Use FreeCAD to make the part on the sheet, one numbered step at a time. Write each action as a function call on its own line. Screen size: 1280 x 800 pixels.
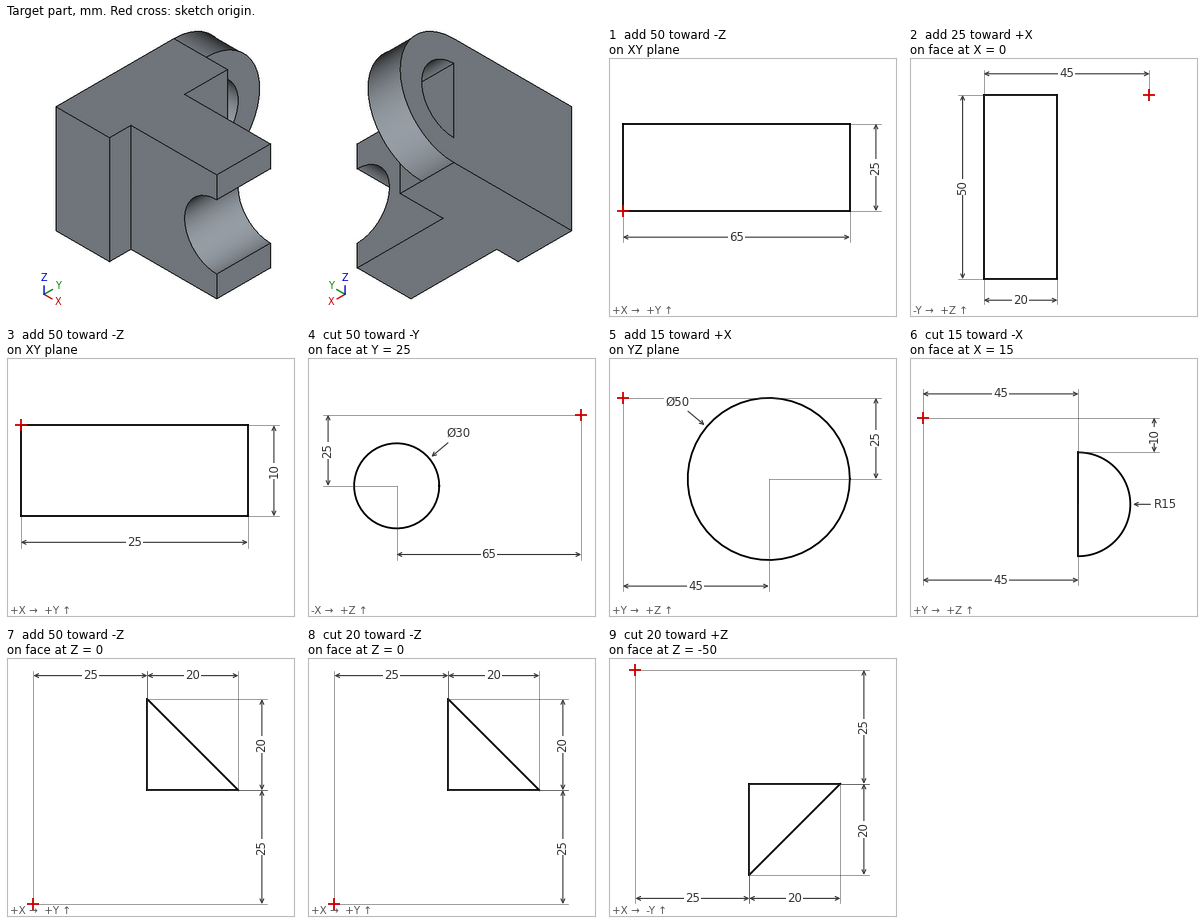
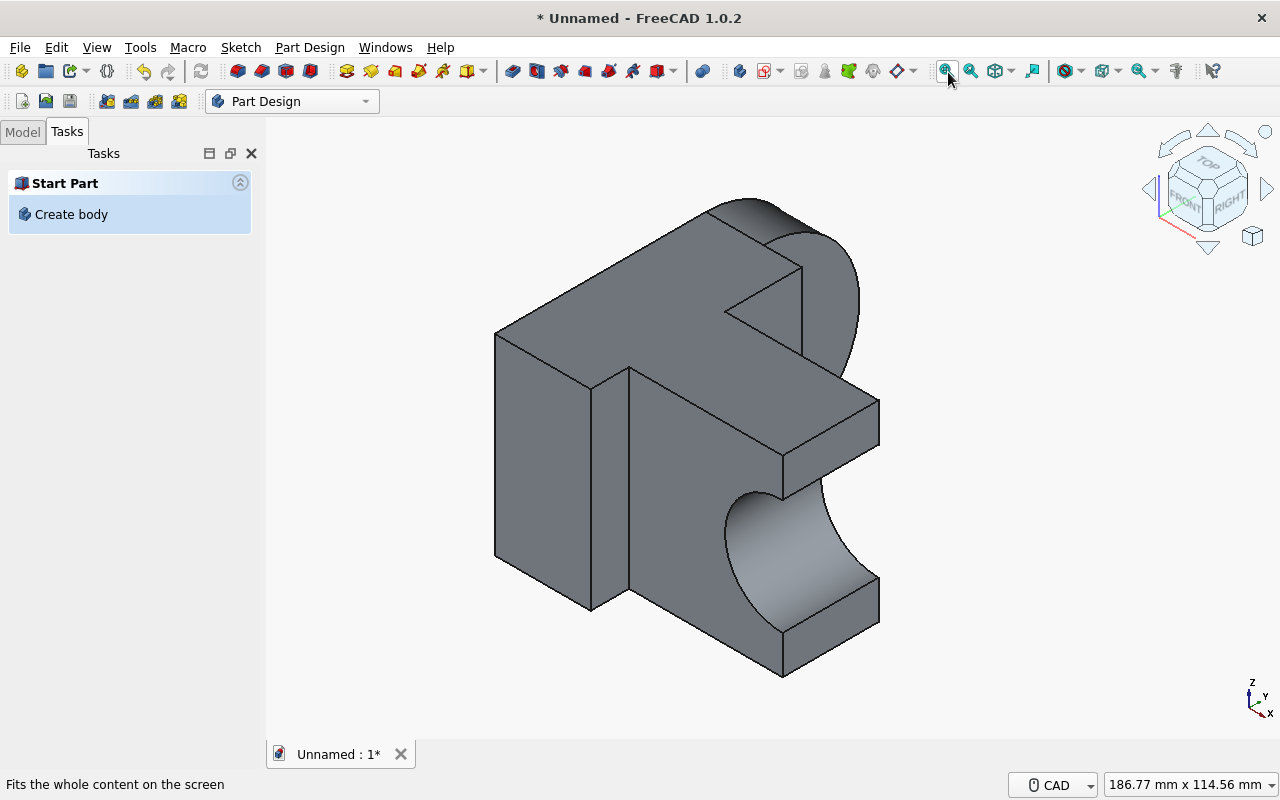
click(811, 327)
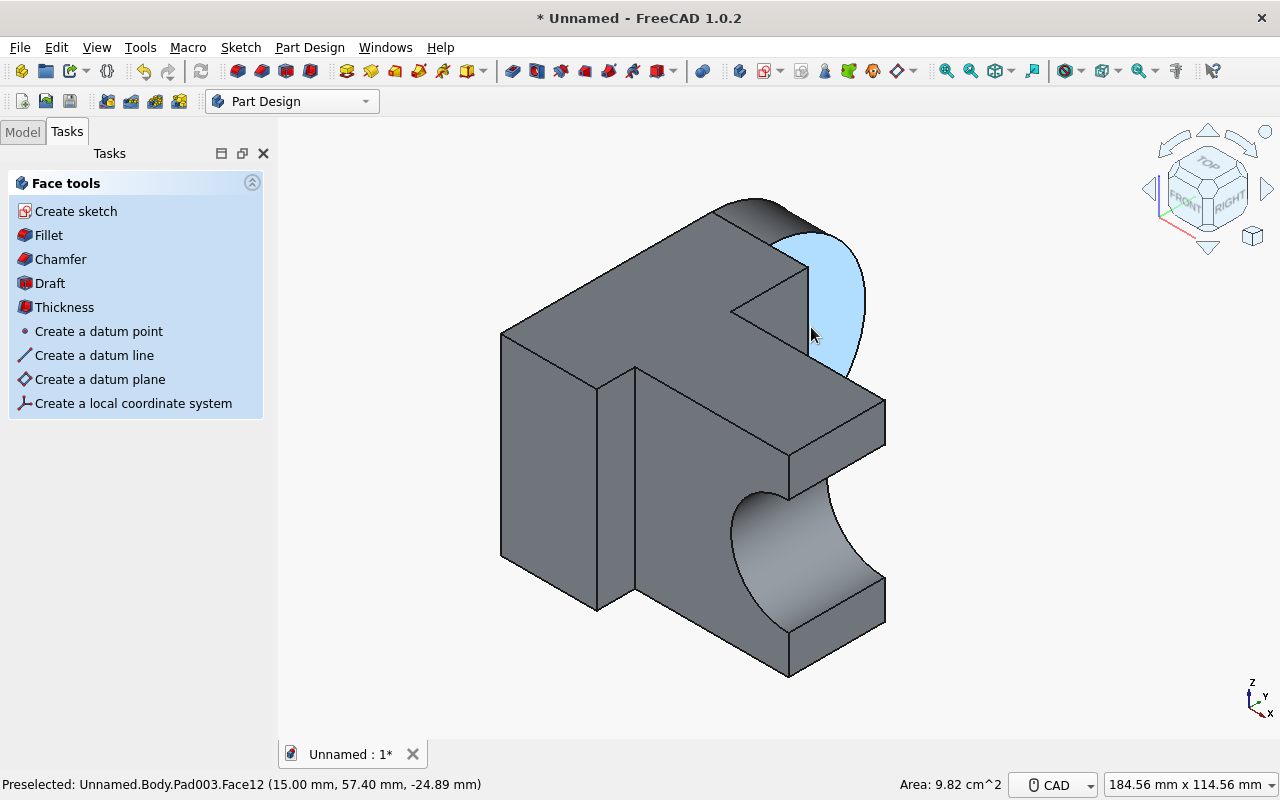
click(764, 72)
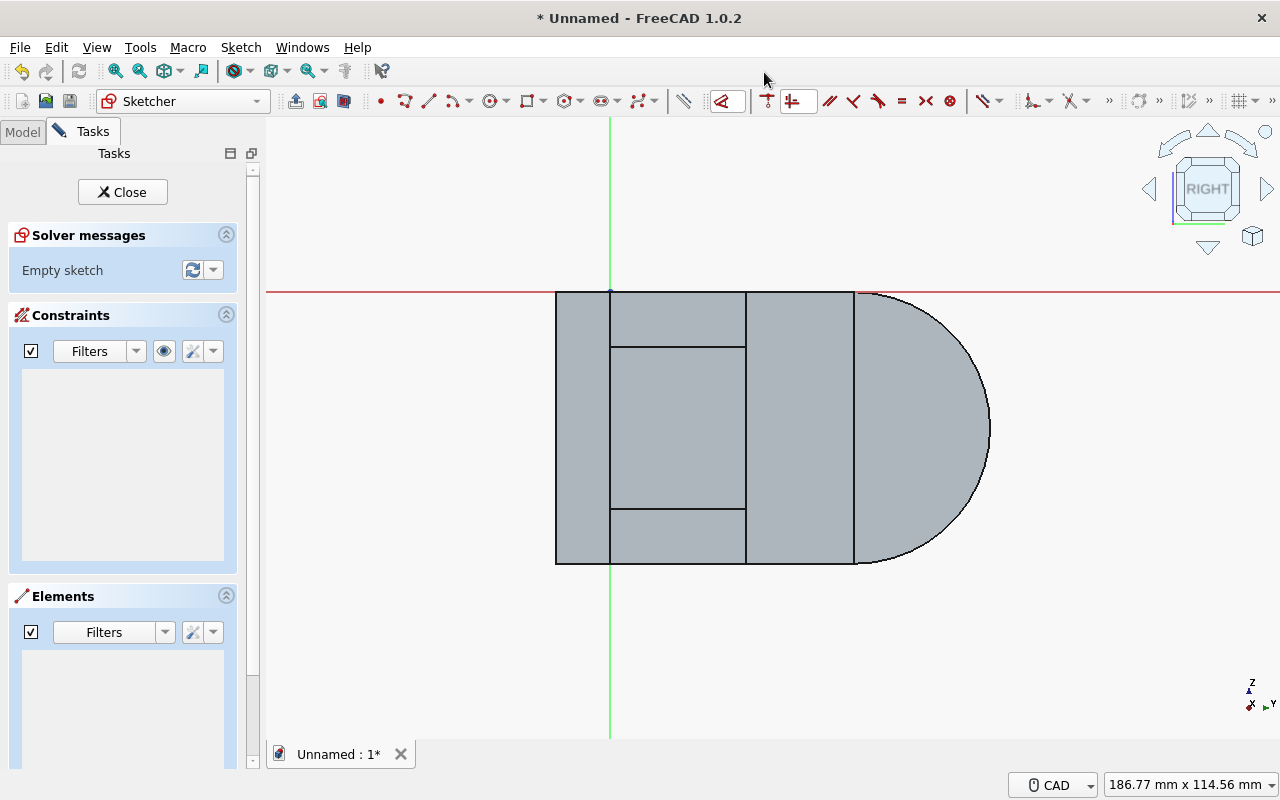
scroll(856, 368, up, 3)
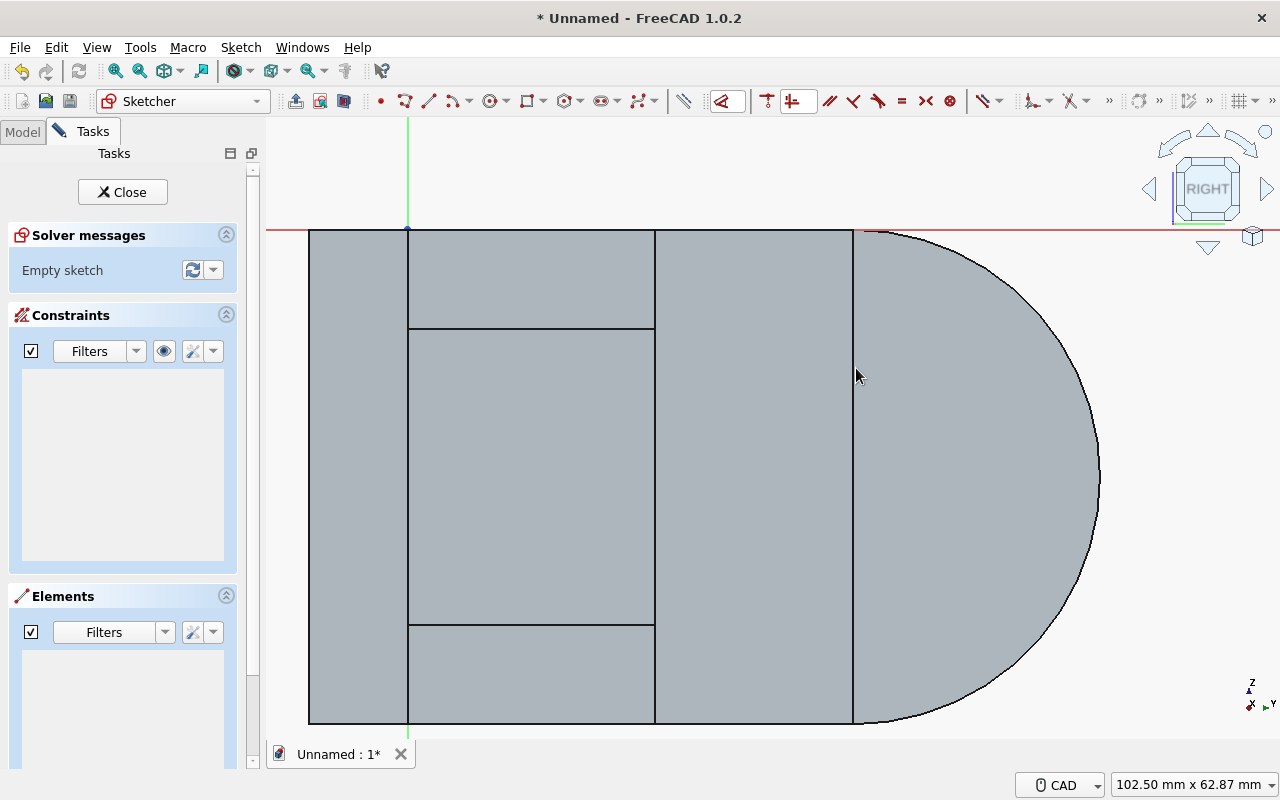
click(430, 102)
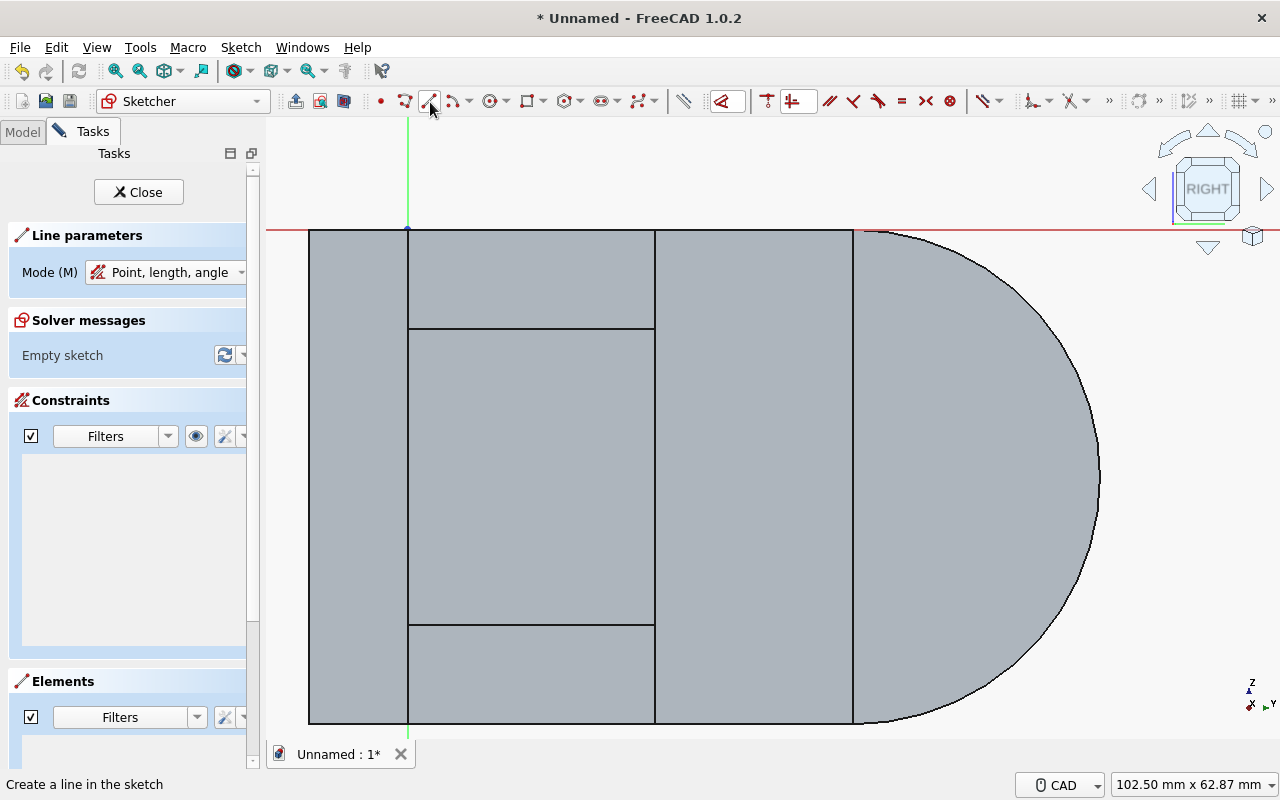
click(853, 329)
click(853, 625)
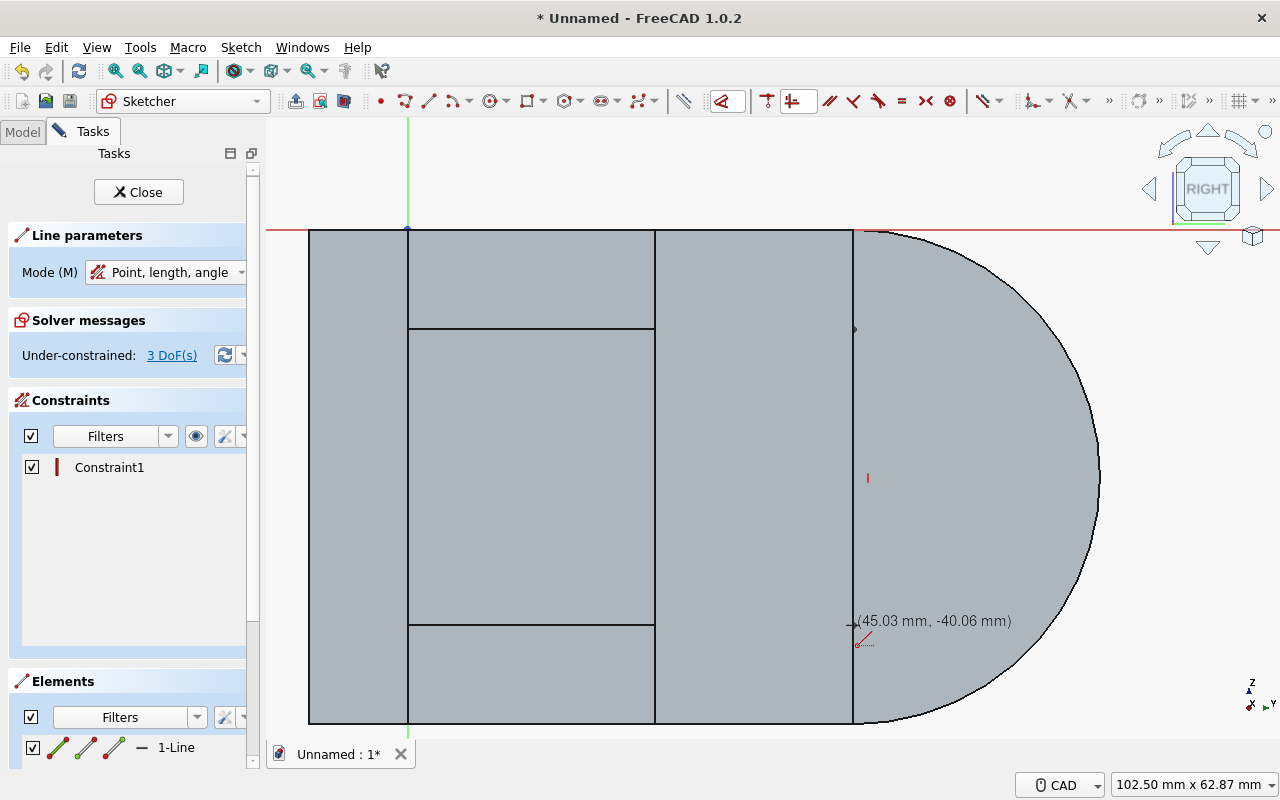
key(g)
key(3)
key(a)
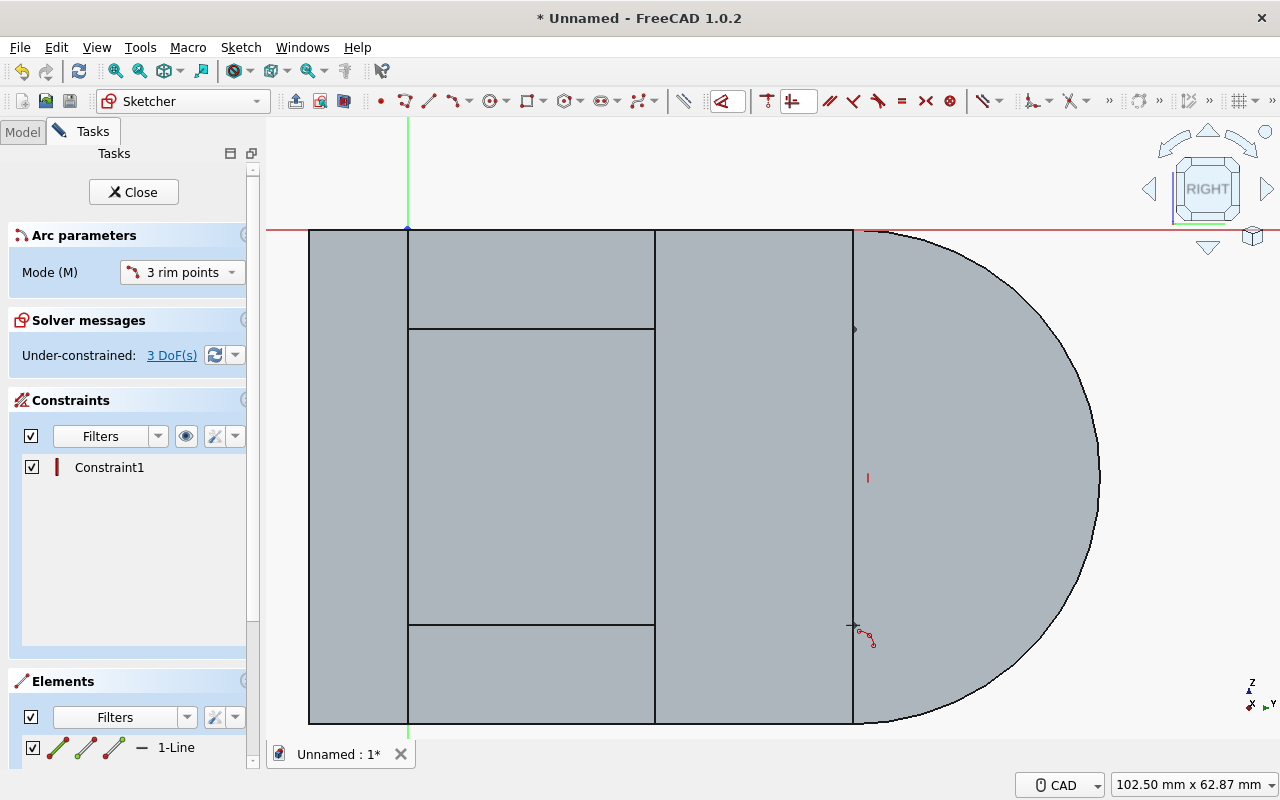
click(853, 626)
click(853, 330)
click(1001, 477)
key(Escape)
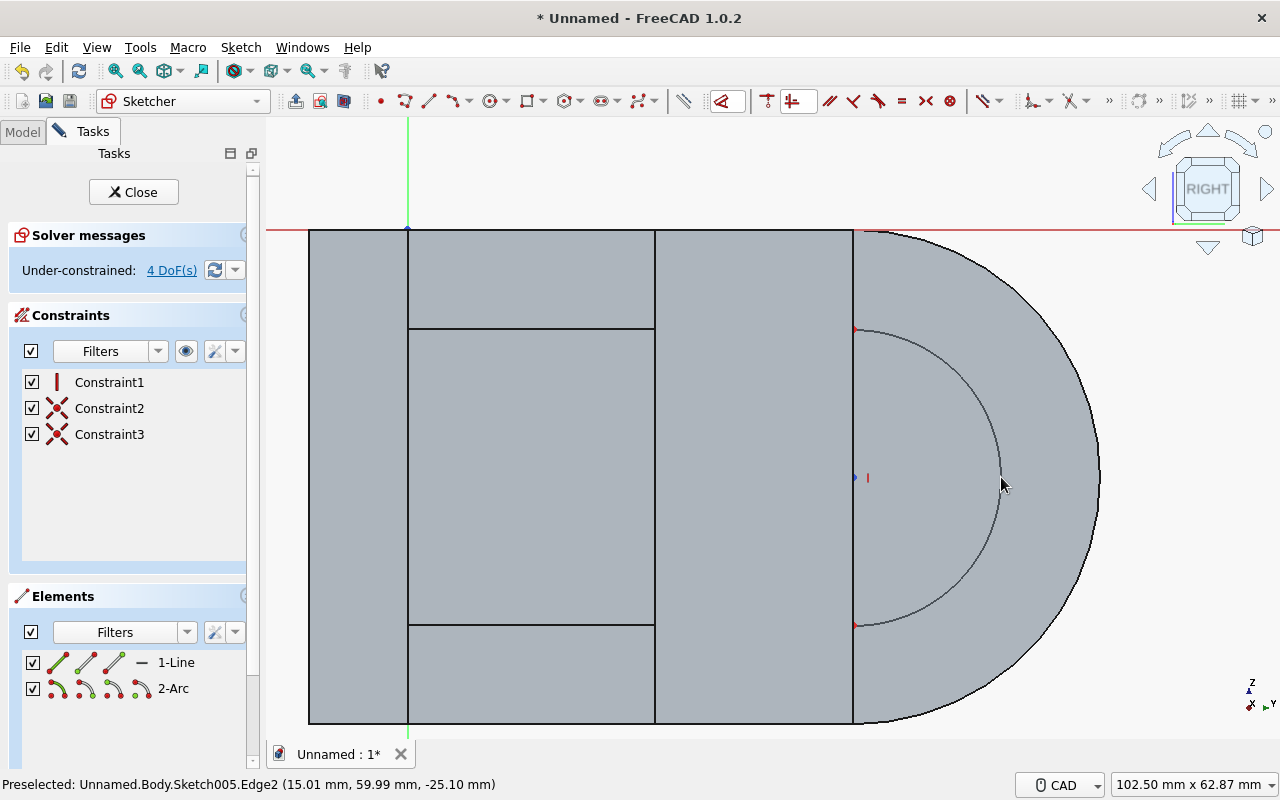
click(973, 565)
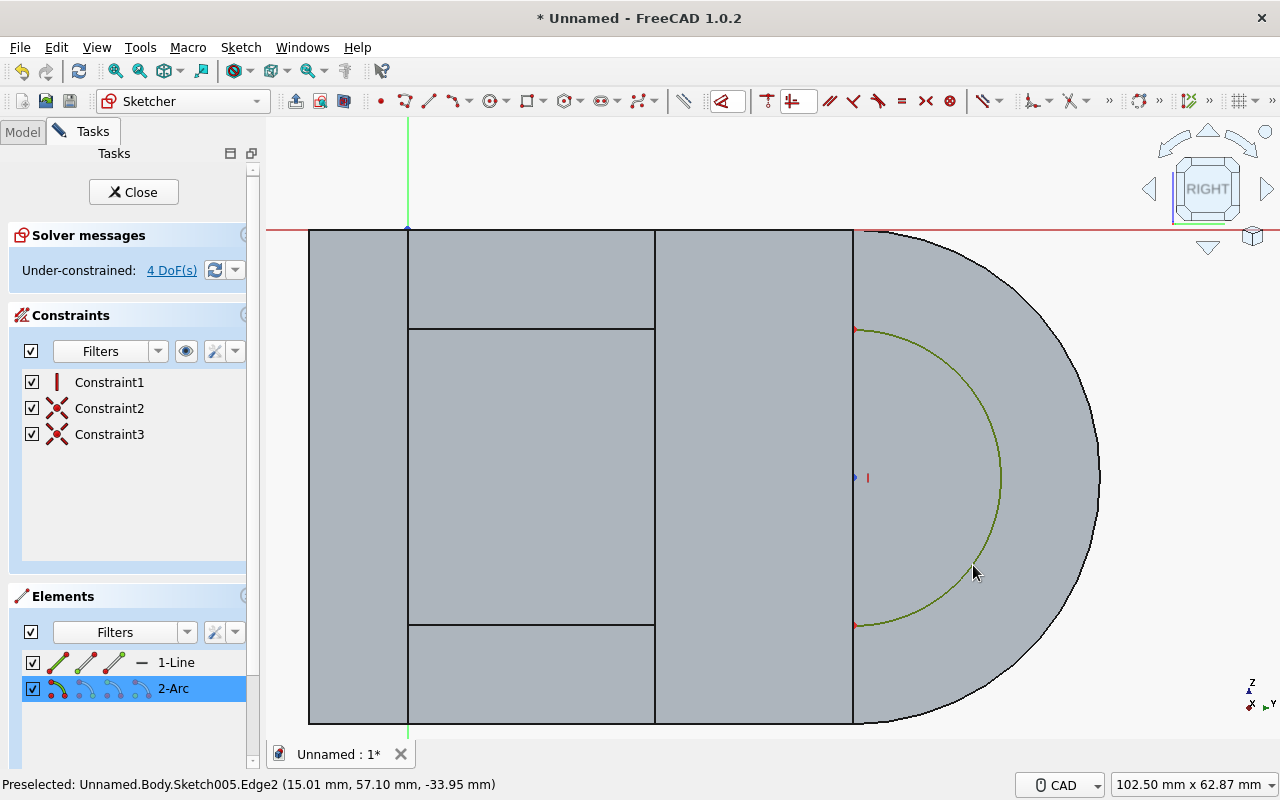
click(740, 102)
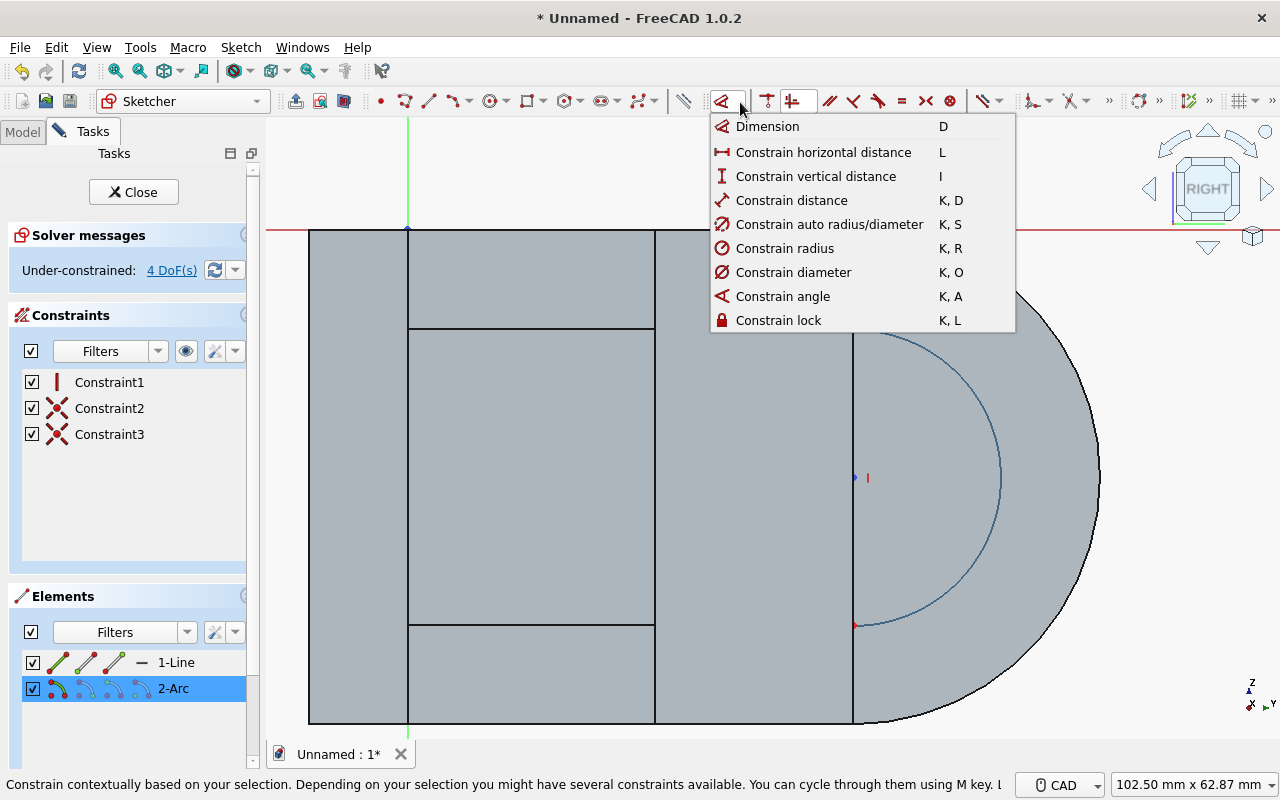
click(863, 248)